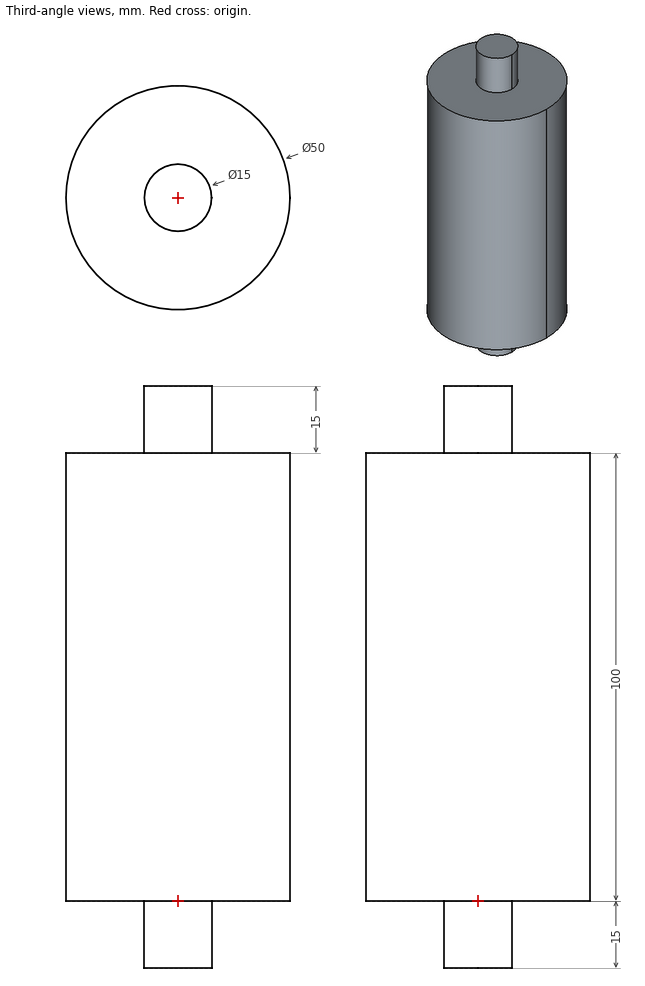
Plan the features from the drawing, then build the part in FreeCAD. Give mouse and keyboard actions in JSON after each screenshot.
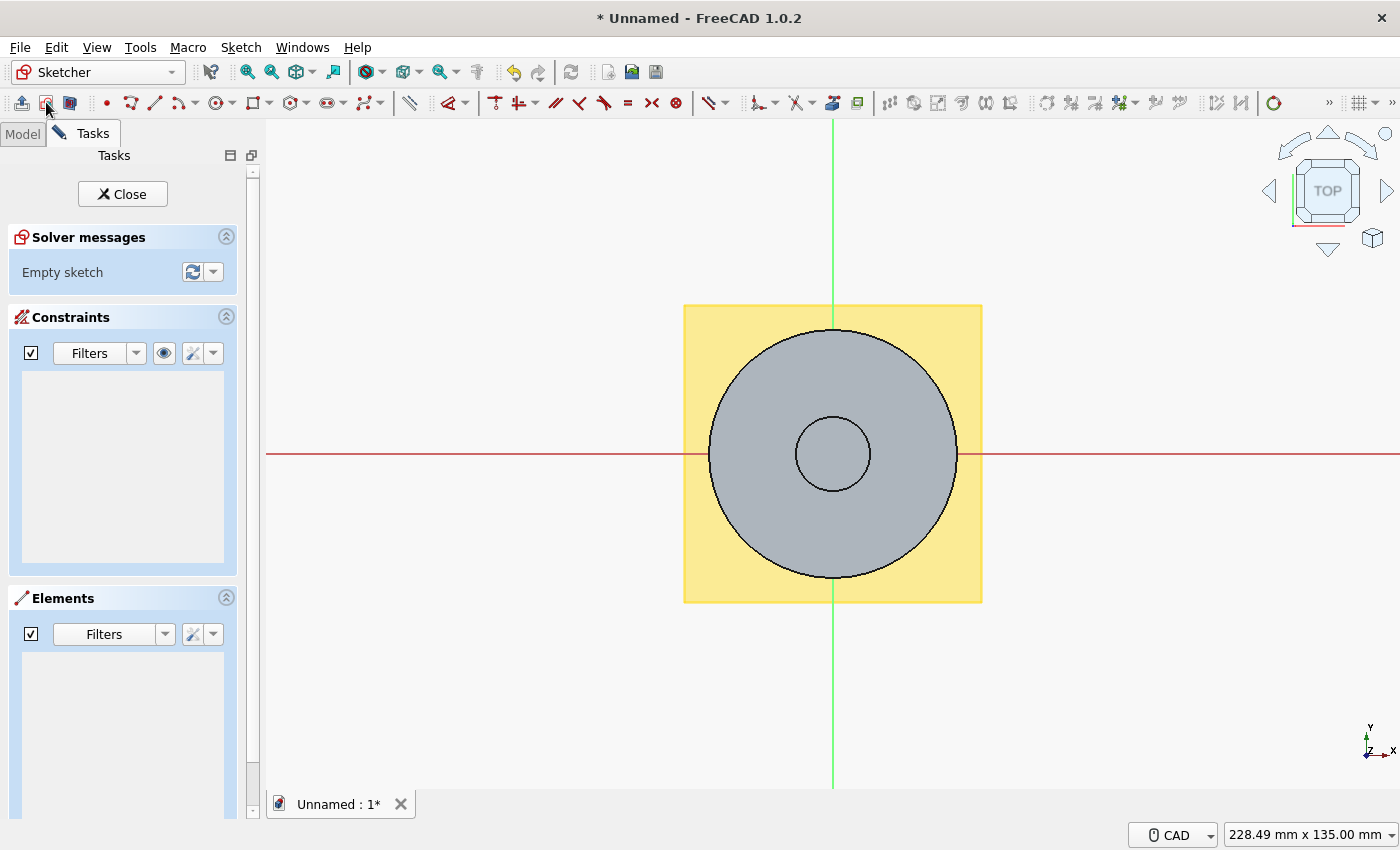
{"action": "left_click", "coordinate": [70, 104]}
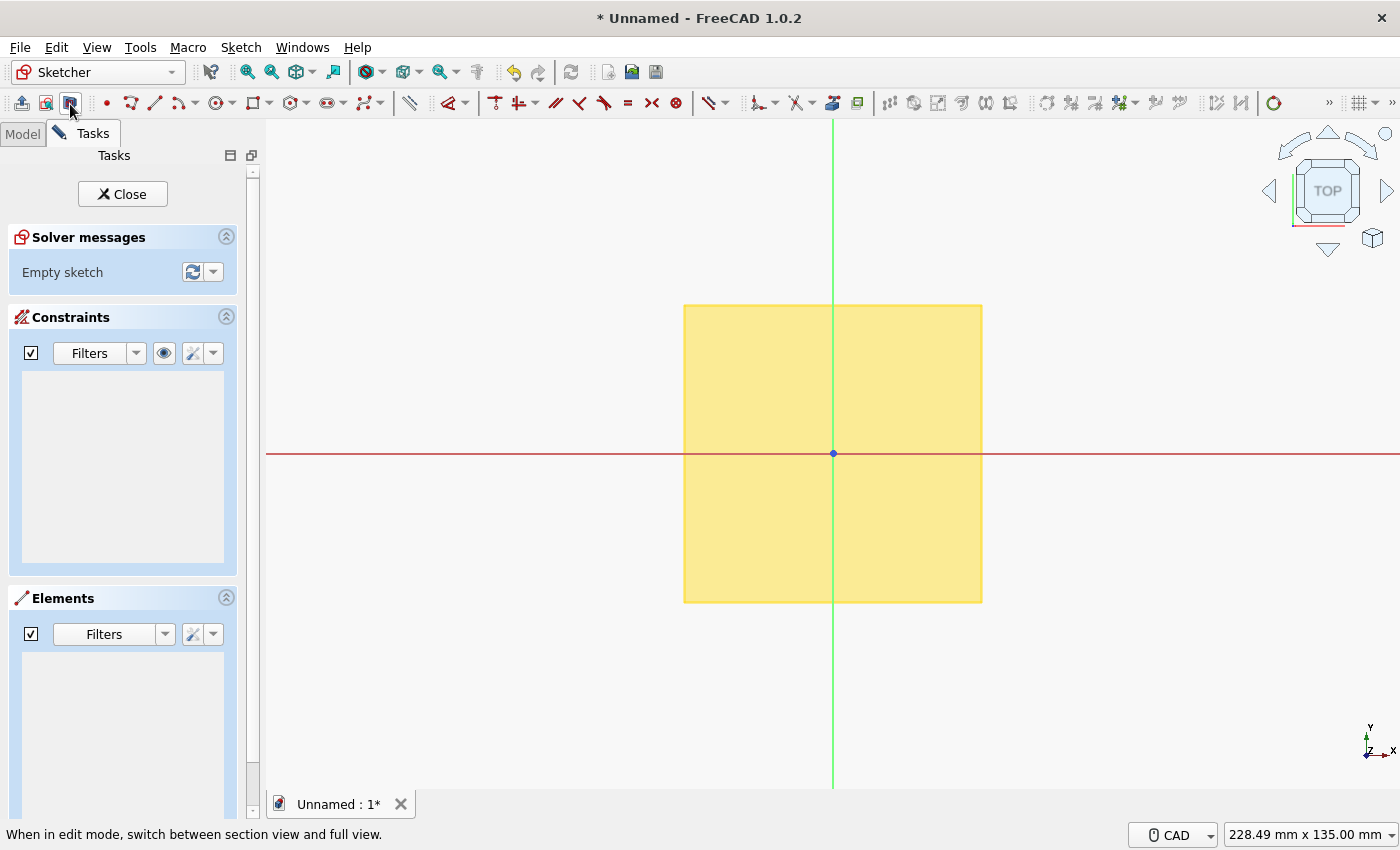
{"action": "scroll", "coordinate": [847, 454], "scroll_direction": "up", "scroll_amount": 9}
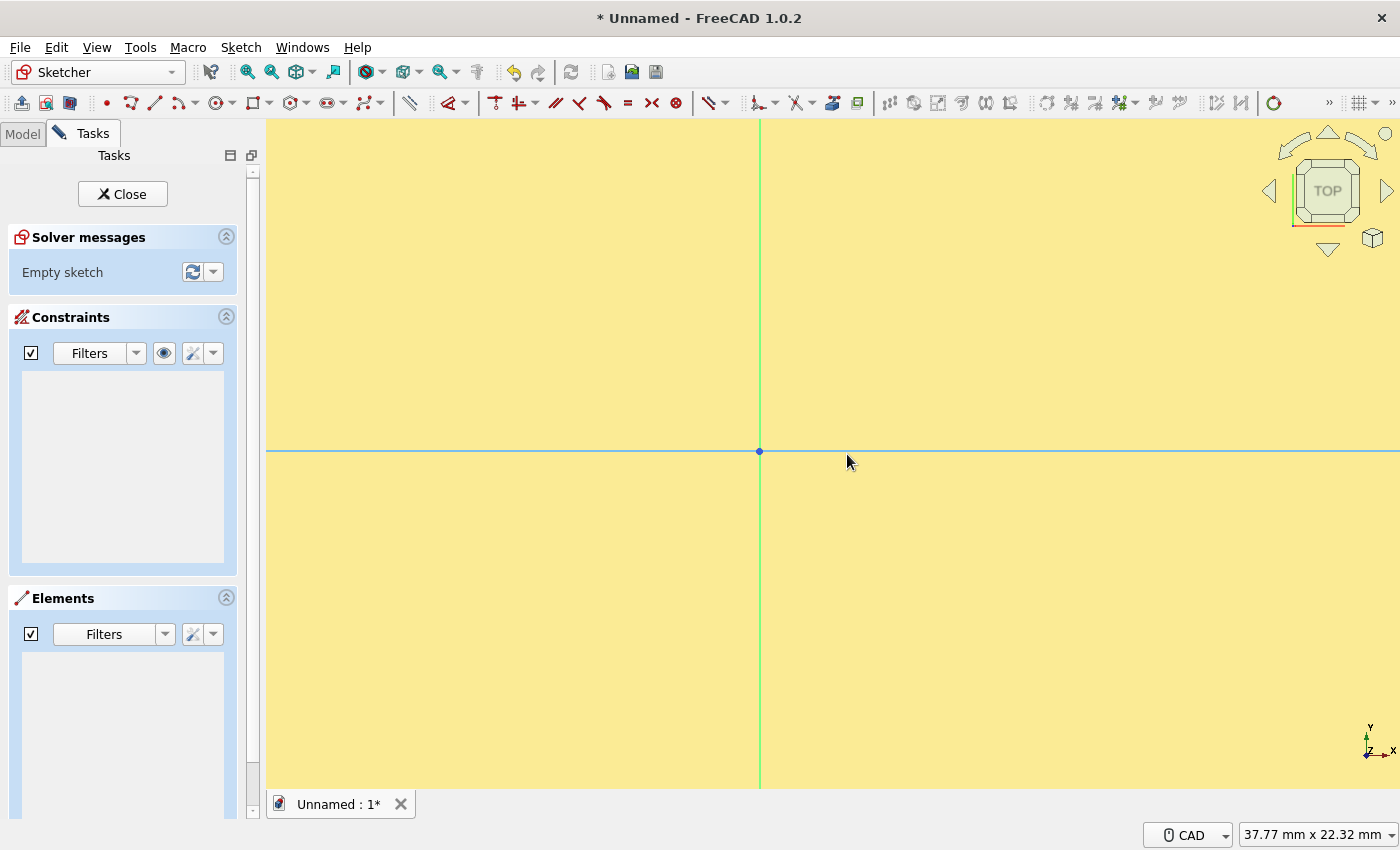
{"action": "left_click", "coordinate": [216, 104]}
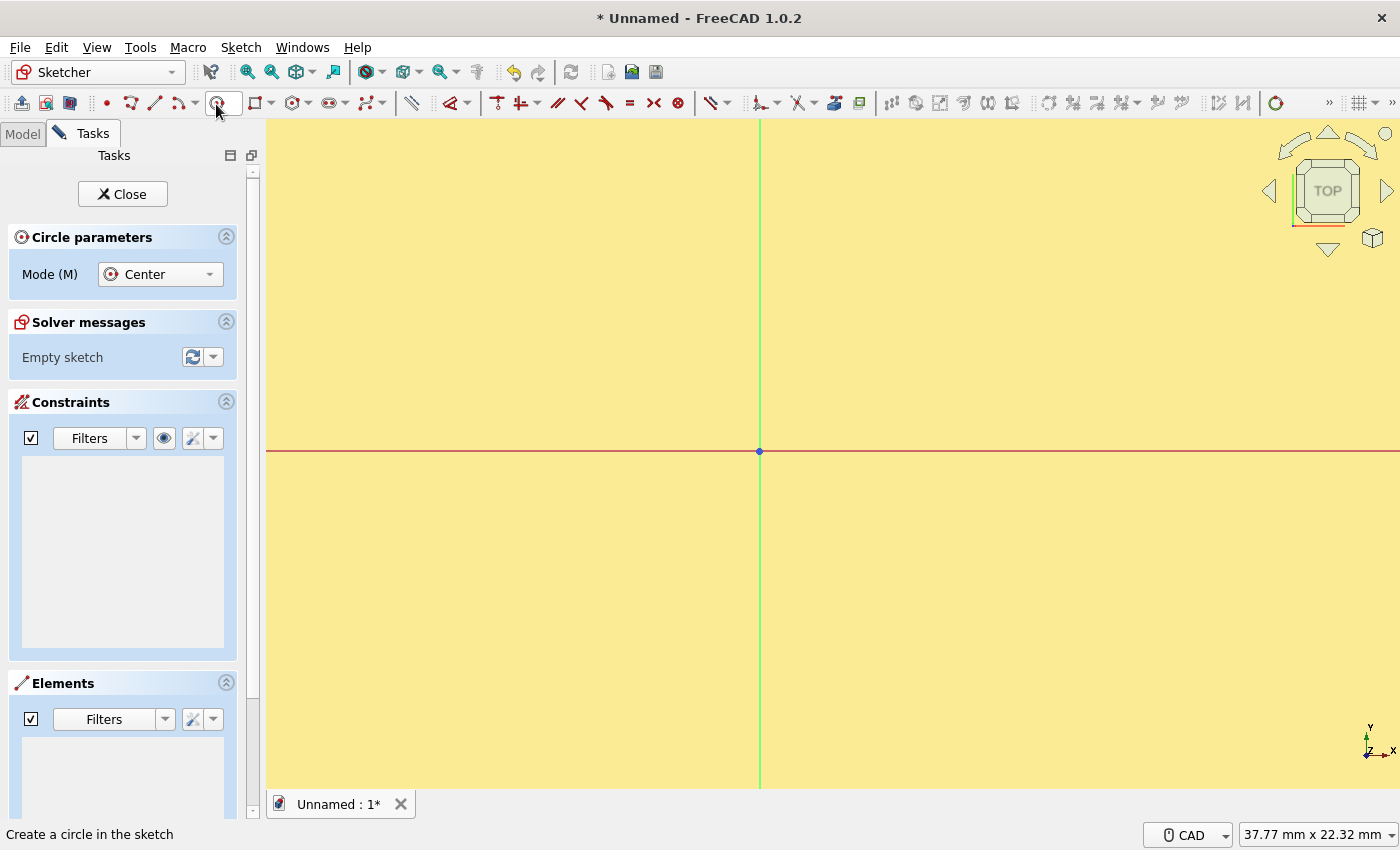
{"action": "left_click", "coordinate": [760, 451]}
{"action": "left_click", "coordinate": [919, 292]}
{"action": "key", "text": "Escape"}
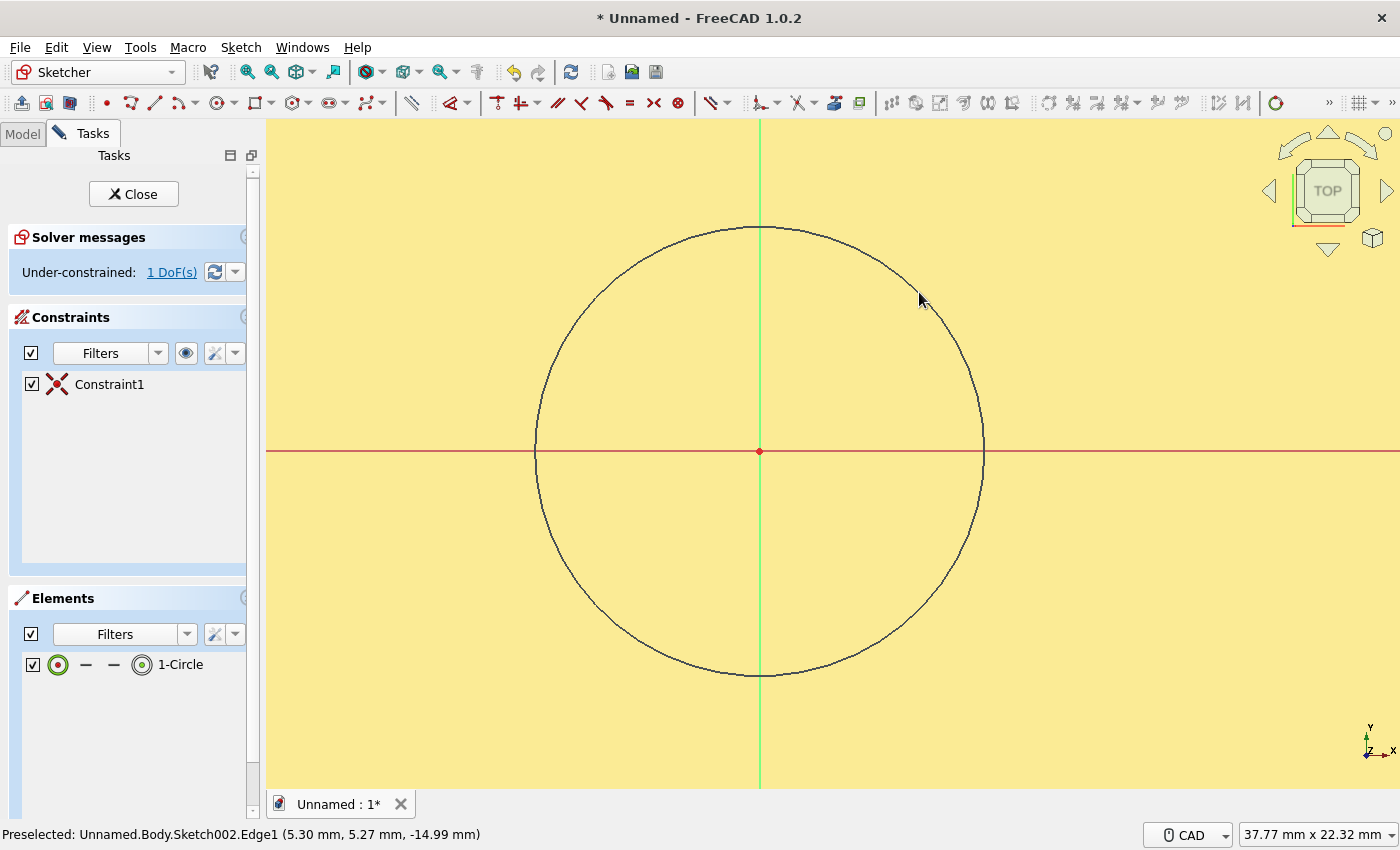
{"action": "left_click", "coordinate": [450, 104]}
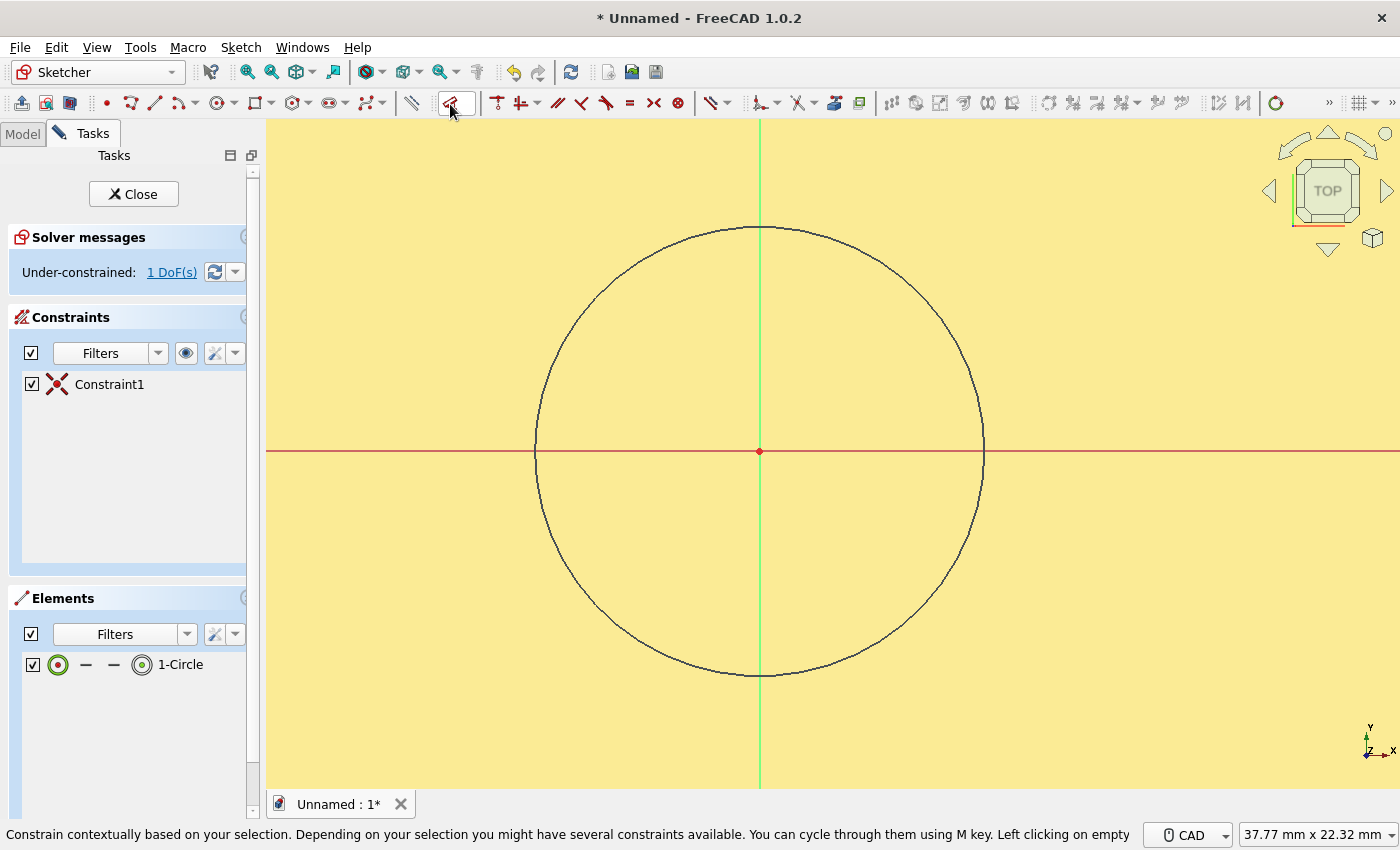
{"action": "left_click", "coordinate": [918, 292]}
{"action": "left_click", "coordinate": [941, 269]}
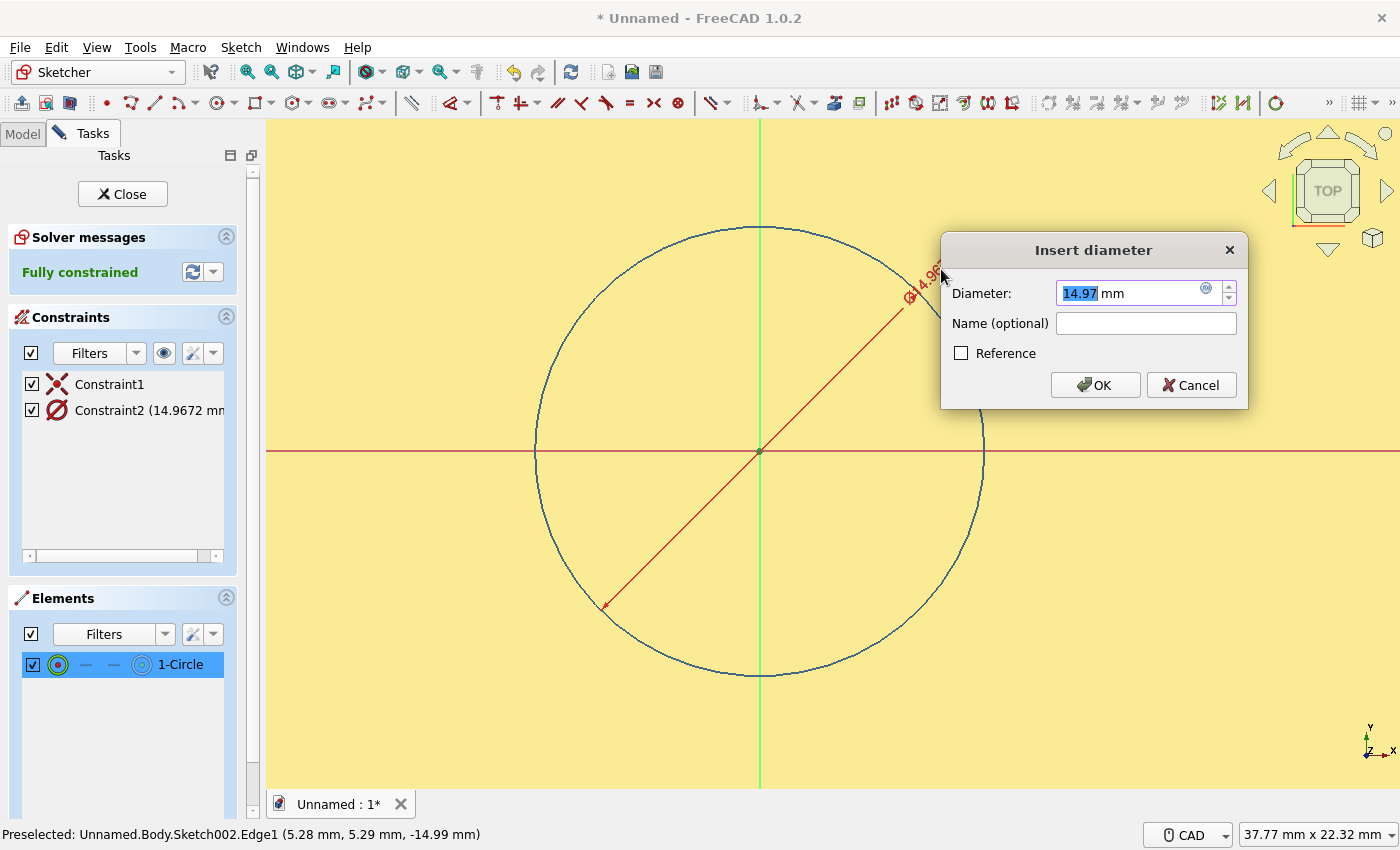
{"action": "type", "text": "15"}
{"action": "key", "text": "Return"}
{"action": "key", "text": "Escape"}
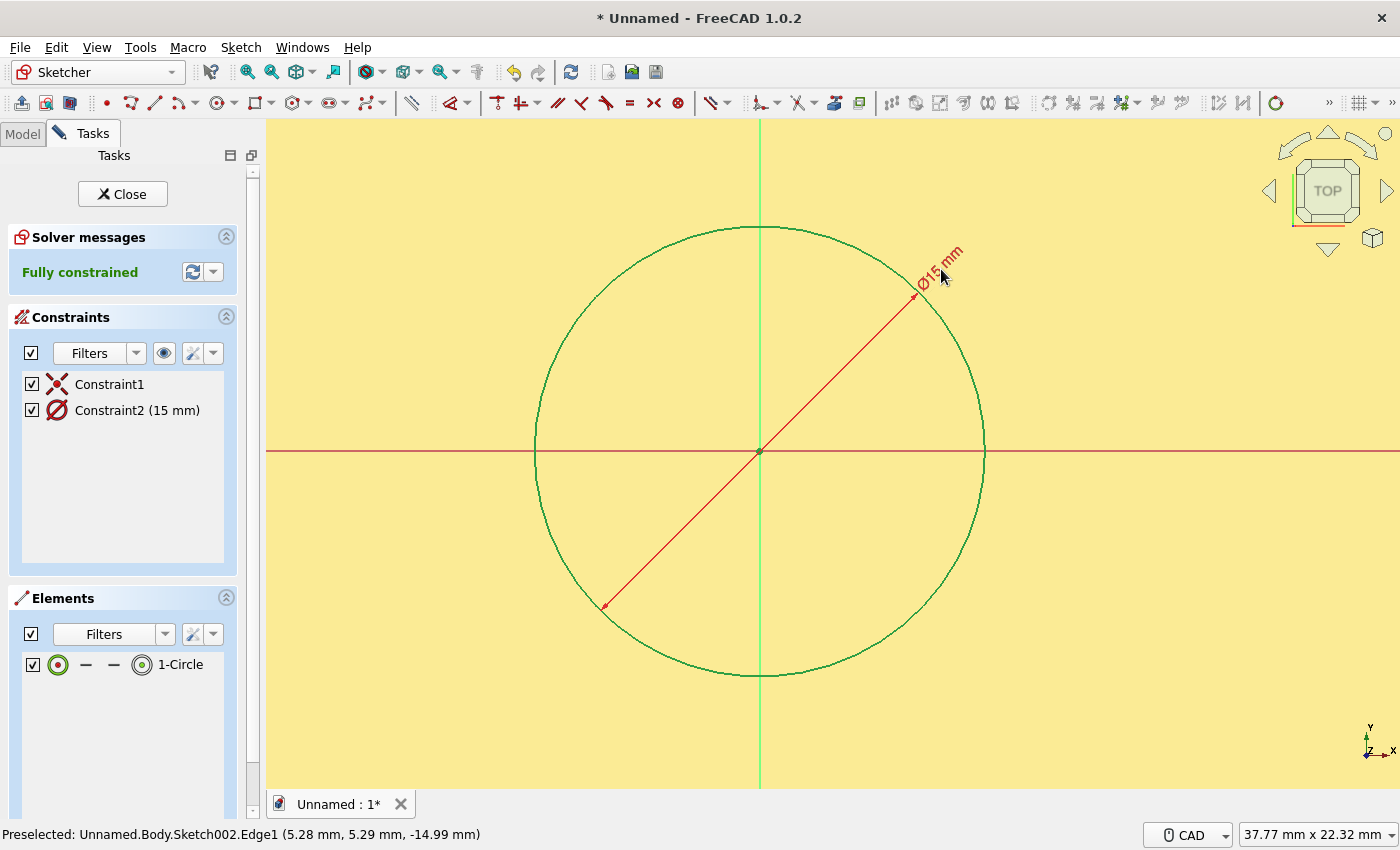
{"action": "left_click", "coordinate": [123, 194]}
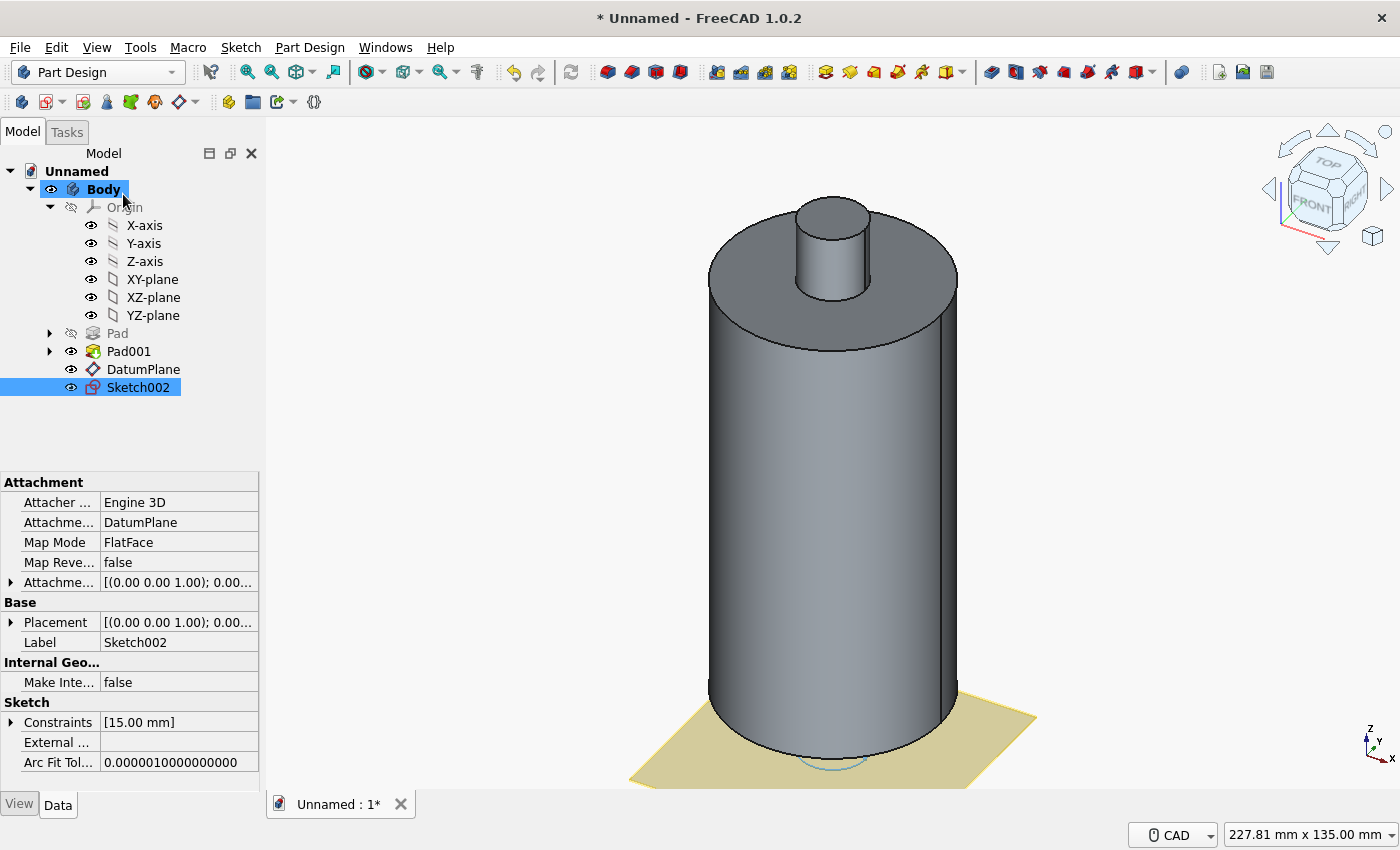
{"action": "left_click", "coordinate": [826, 72]}